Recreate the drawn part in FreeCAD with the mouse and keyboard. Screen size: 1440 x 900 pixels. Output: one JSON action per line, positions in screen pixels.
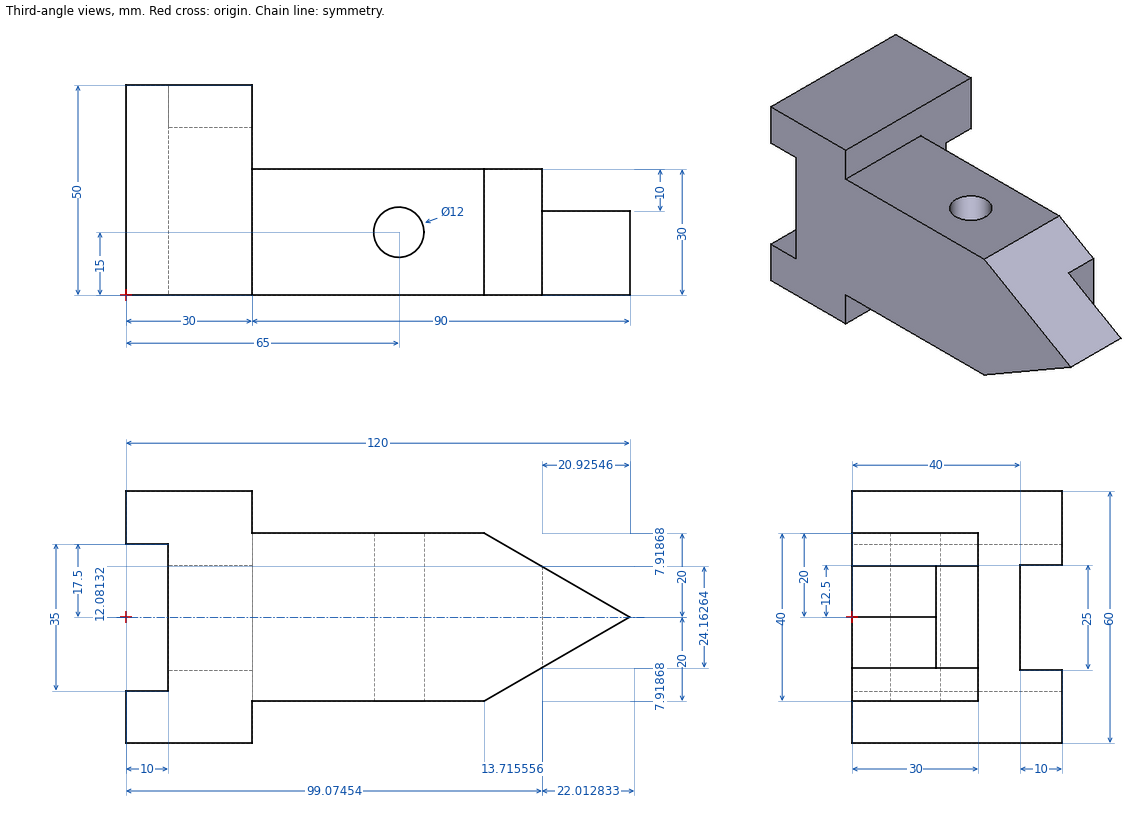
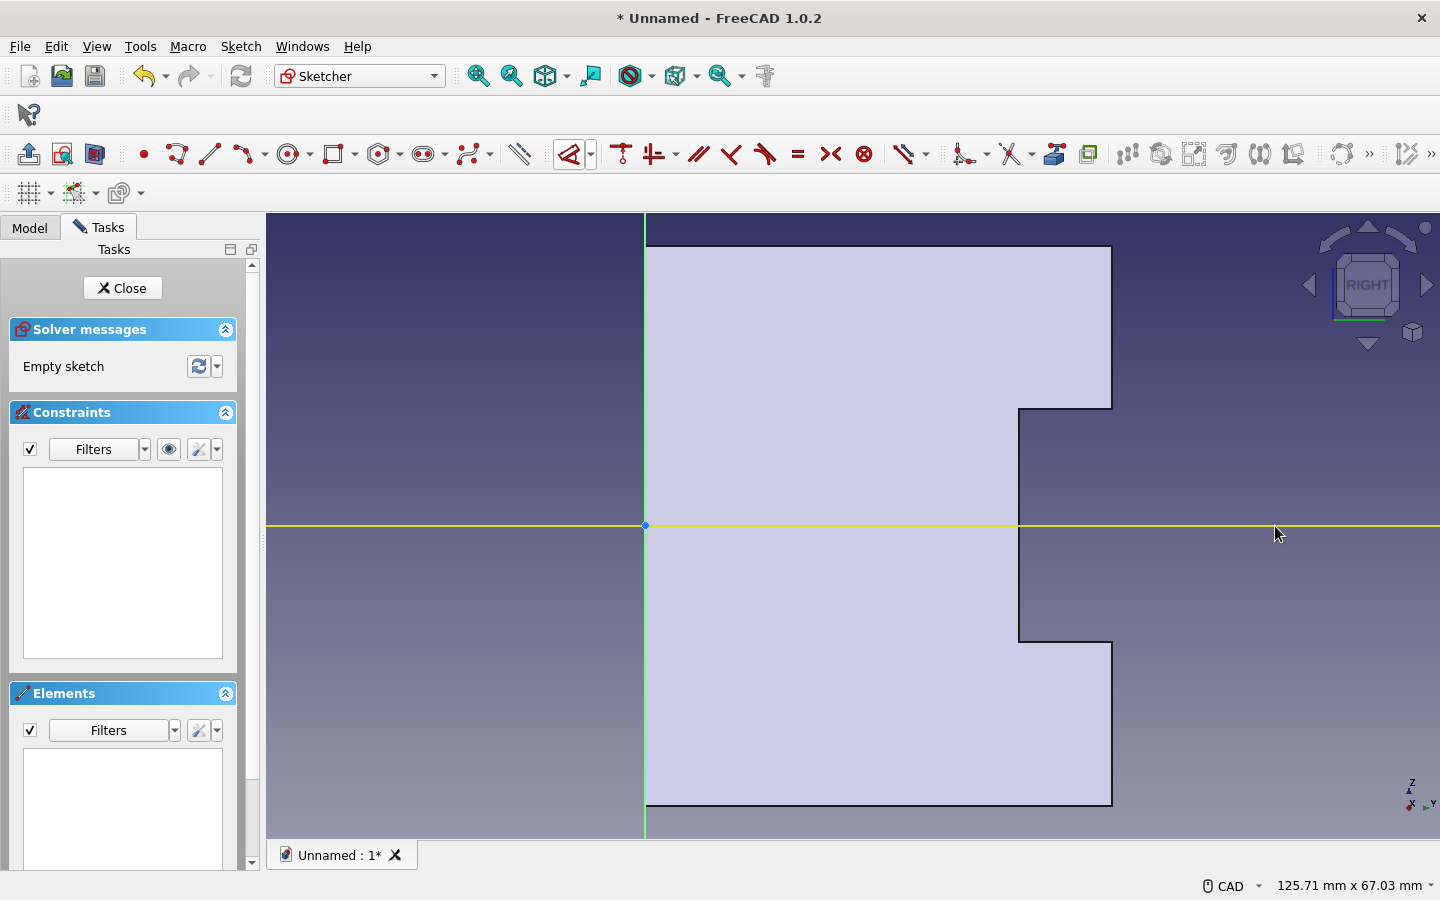
{"action": "left_click", "coordinate": [332, 154]}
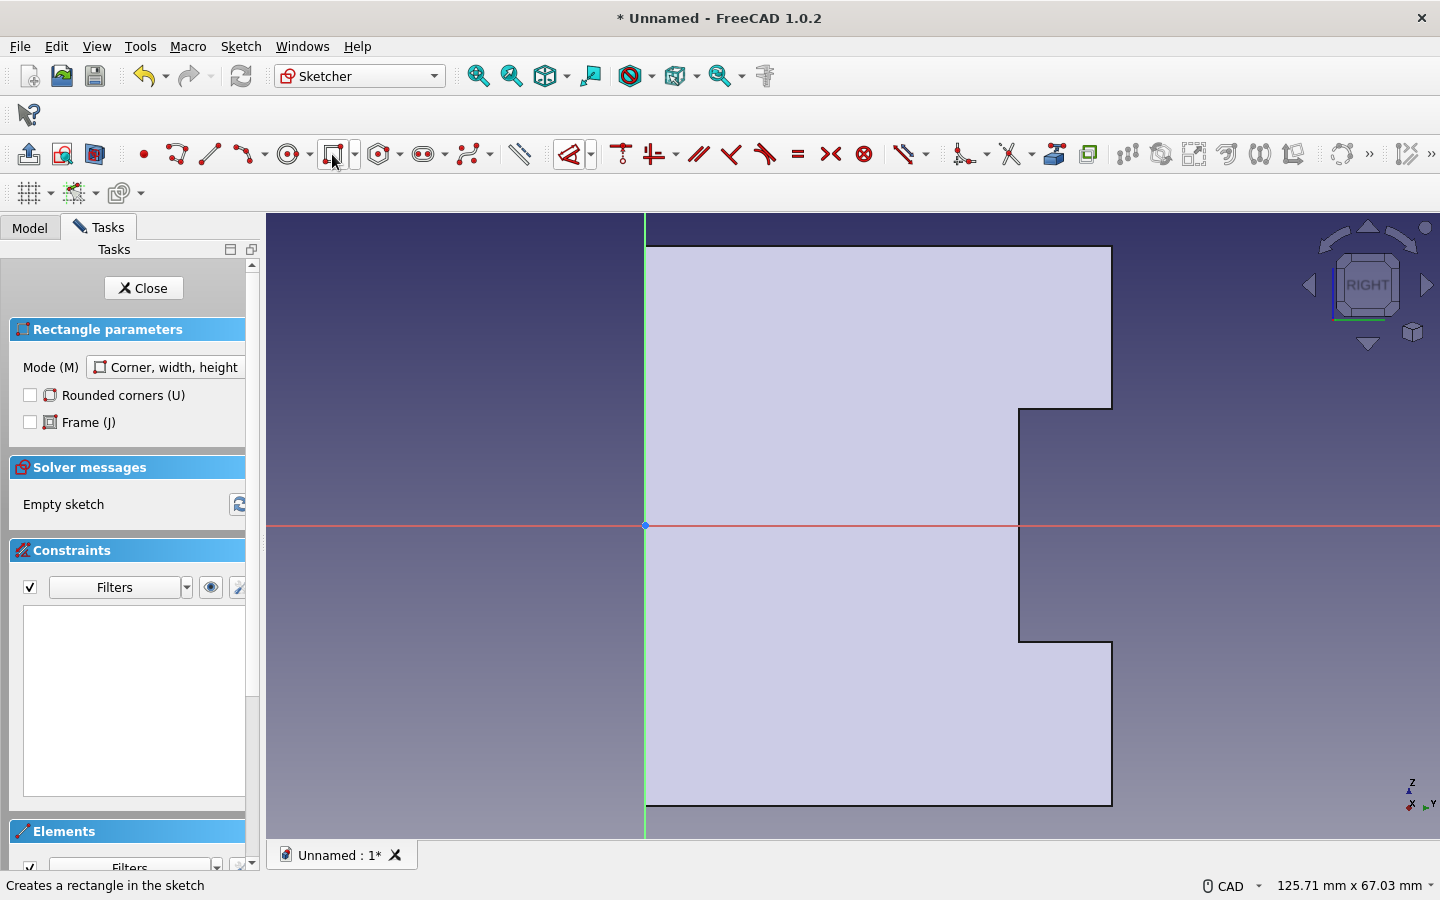
{"action": "left_click", "coordinate": [645, 339]}
{"action": "left_click", "coordinate": [925, 713]}
{"action": "key", "text": "Escape"}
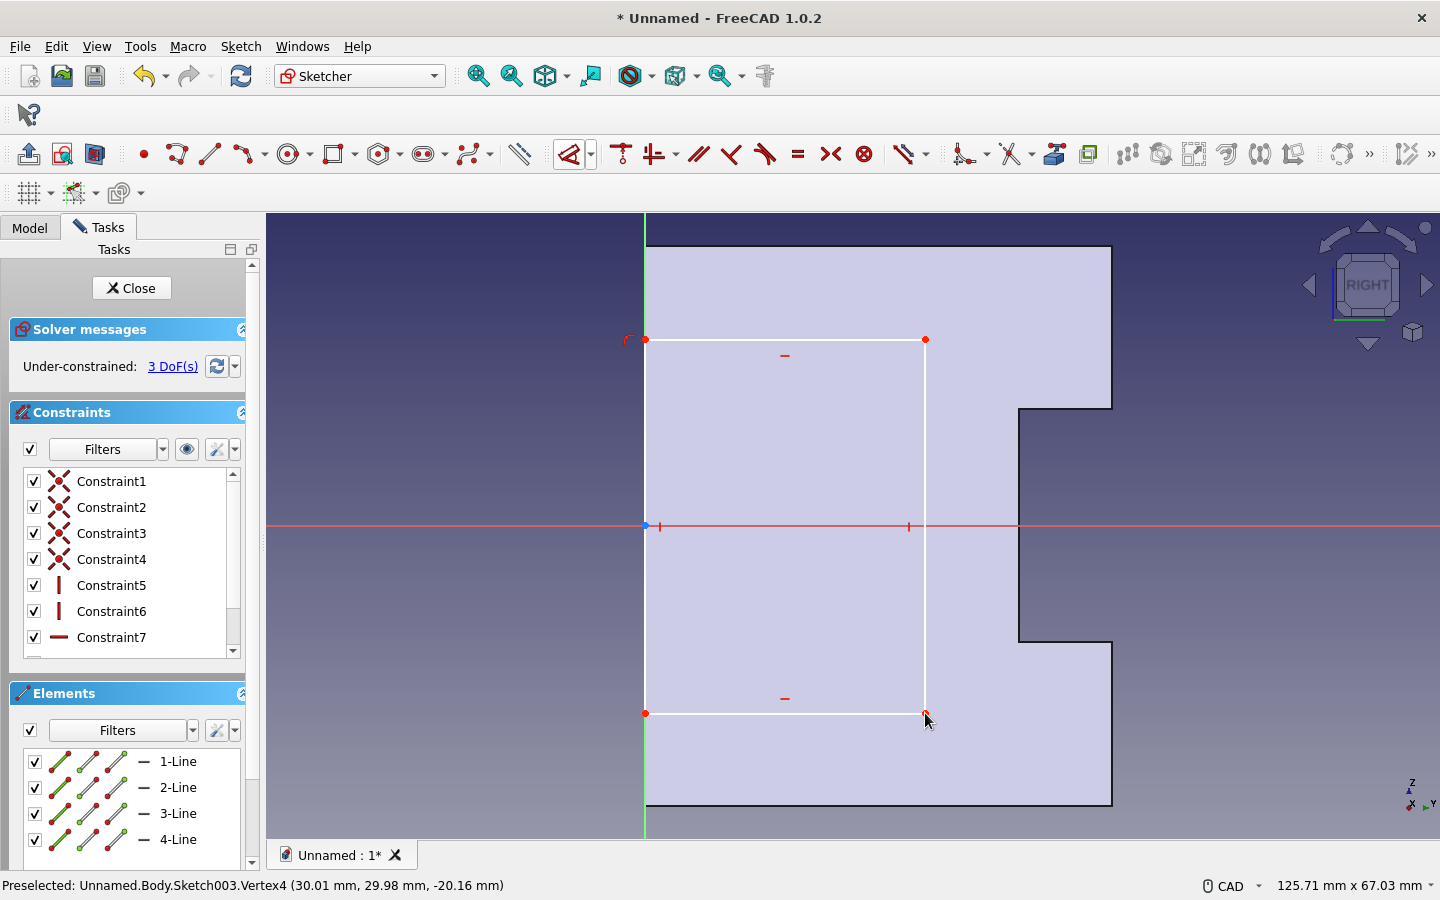
{"action": "left_click", "coordinate": [645, 452]}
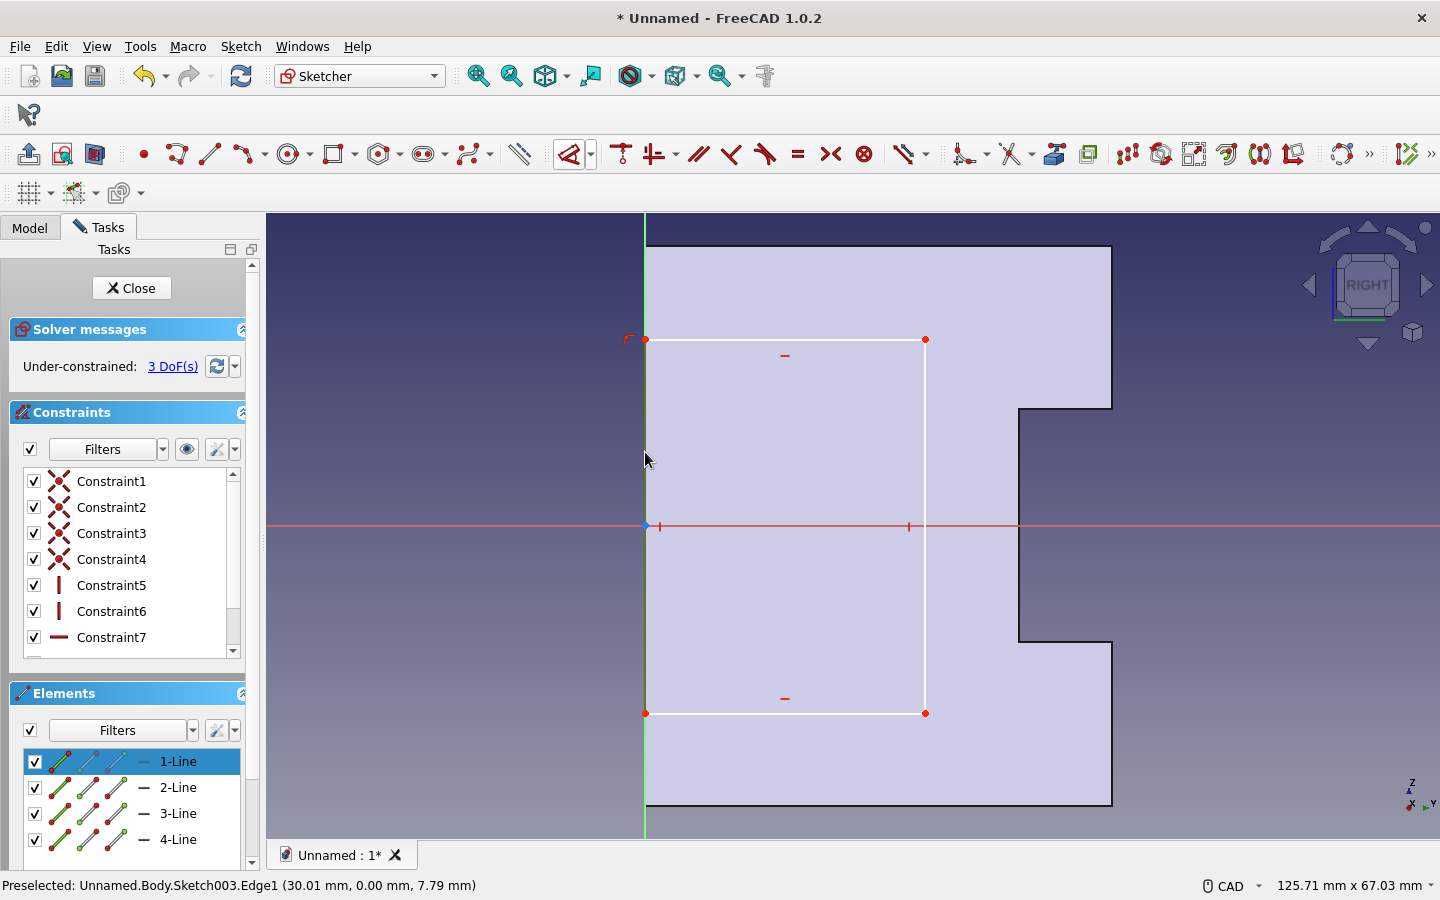
{"action": "left_click", "coordinate": [590, 154]}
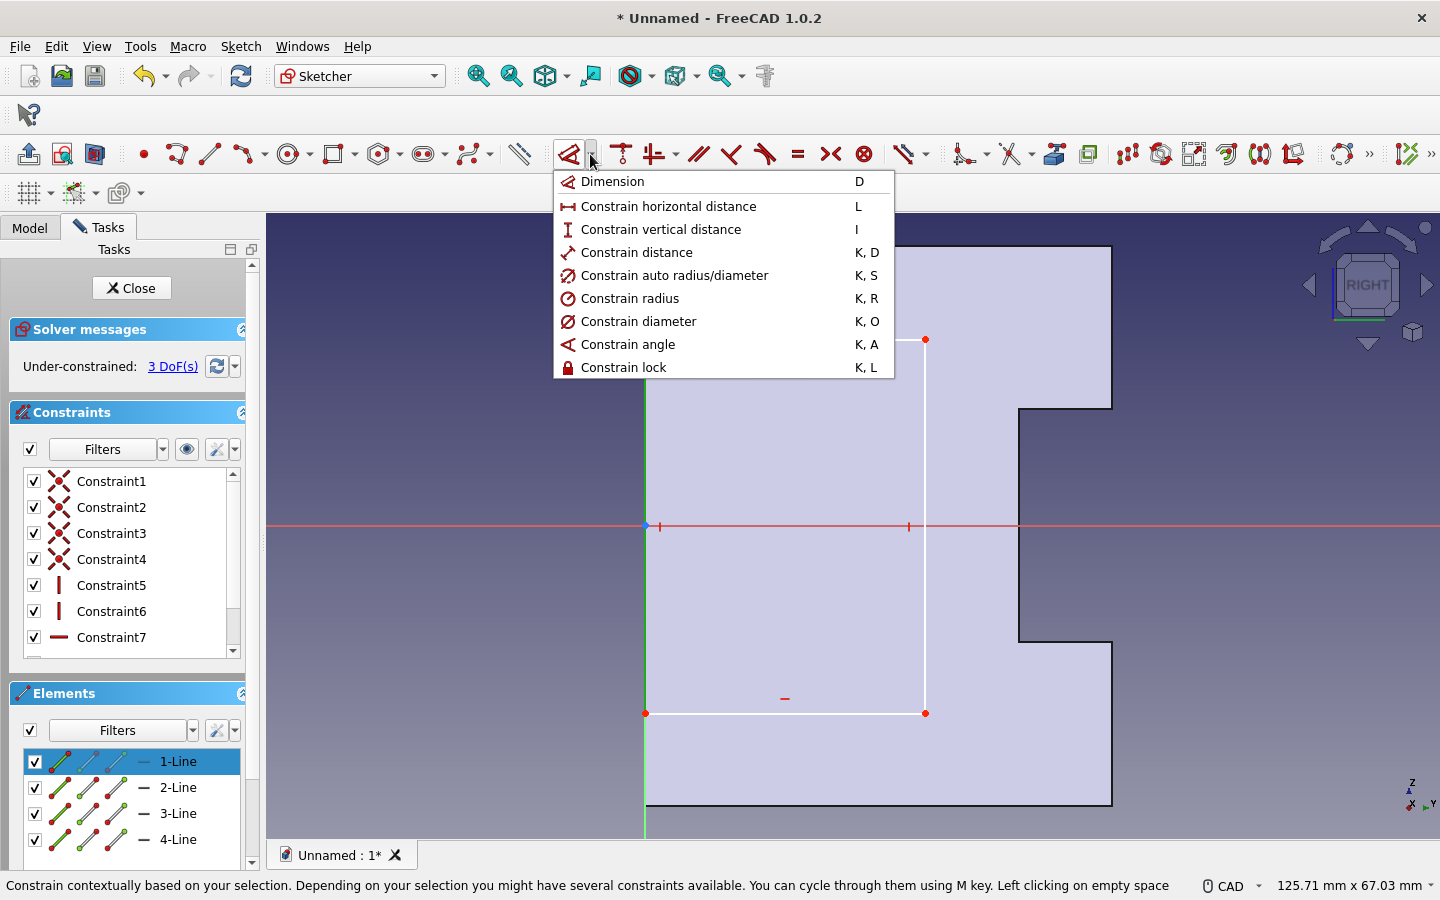
{"action": "left_click", "coordinate": [724, 230]}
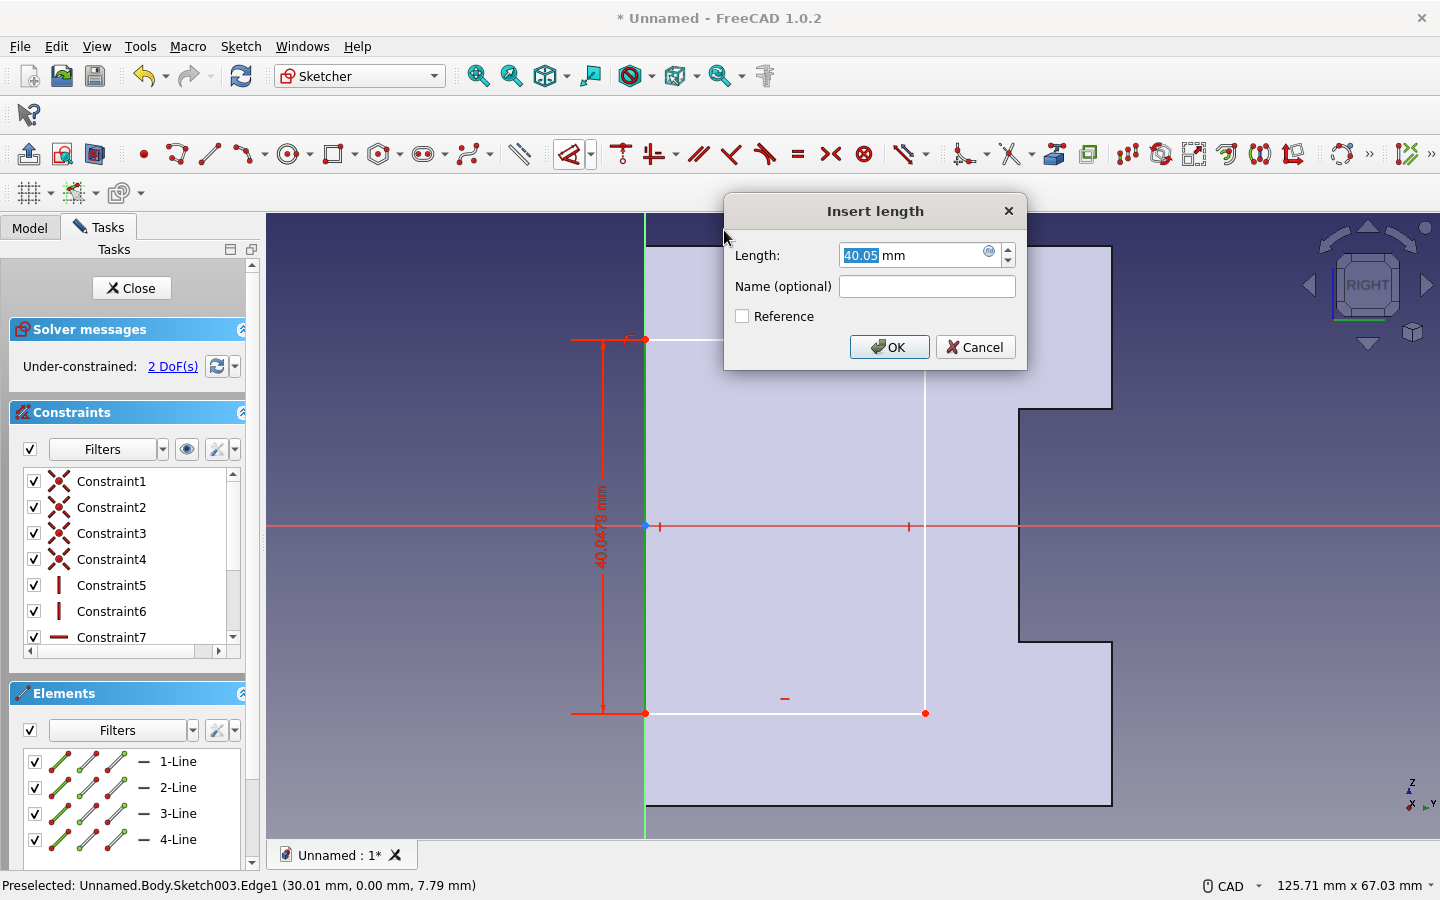
{"action": "type", "text": "40"}
{"action": "key", "text": "Return"}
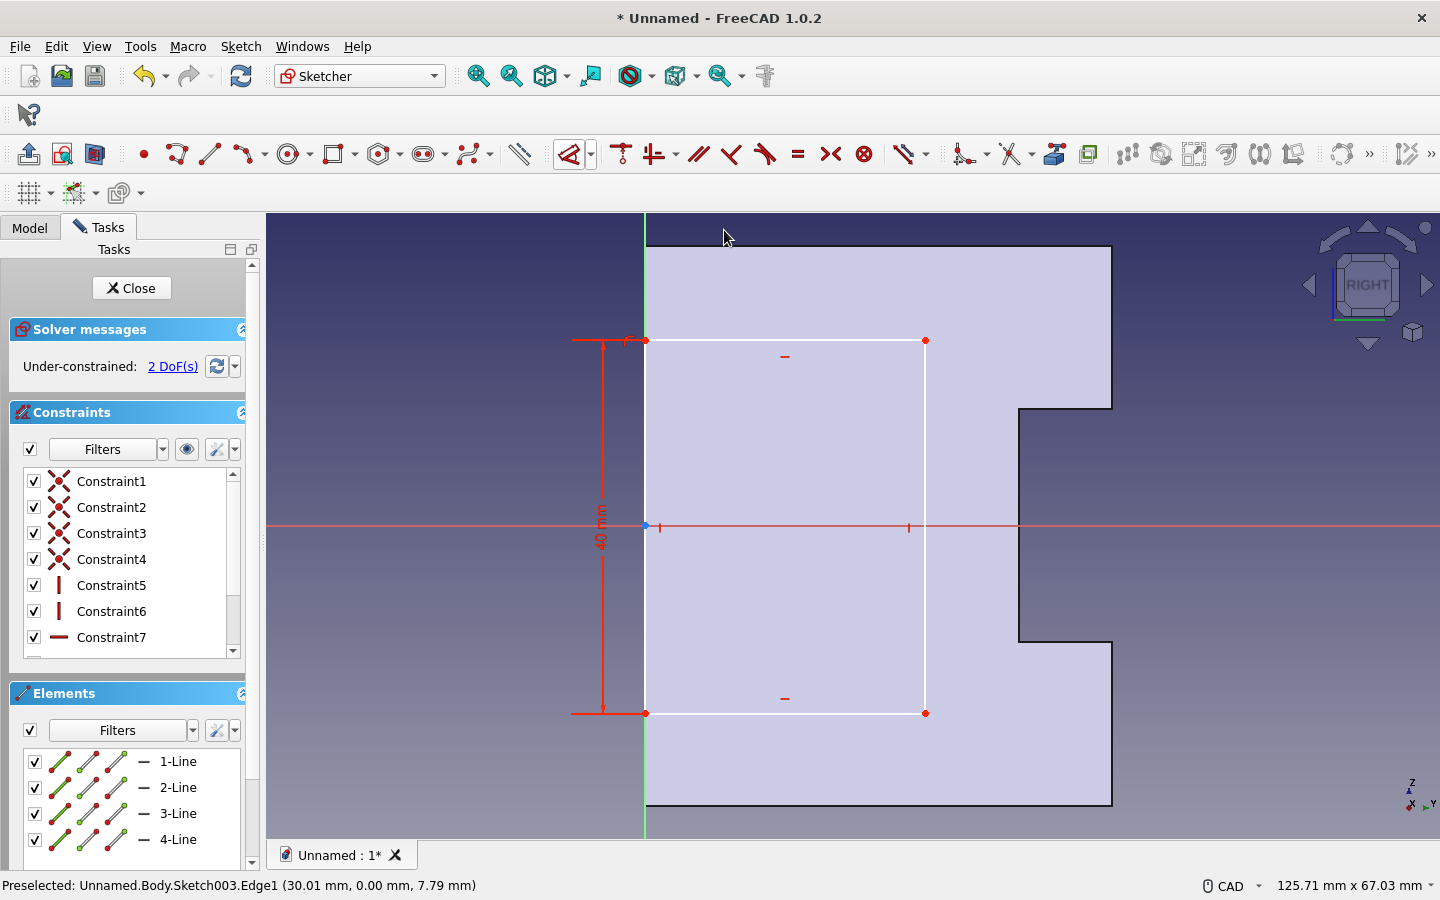
{"action": "left_click", "coordinate": [729, 714]}